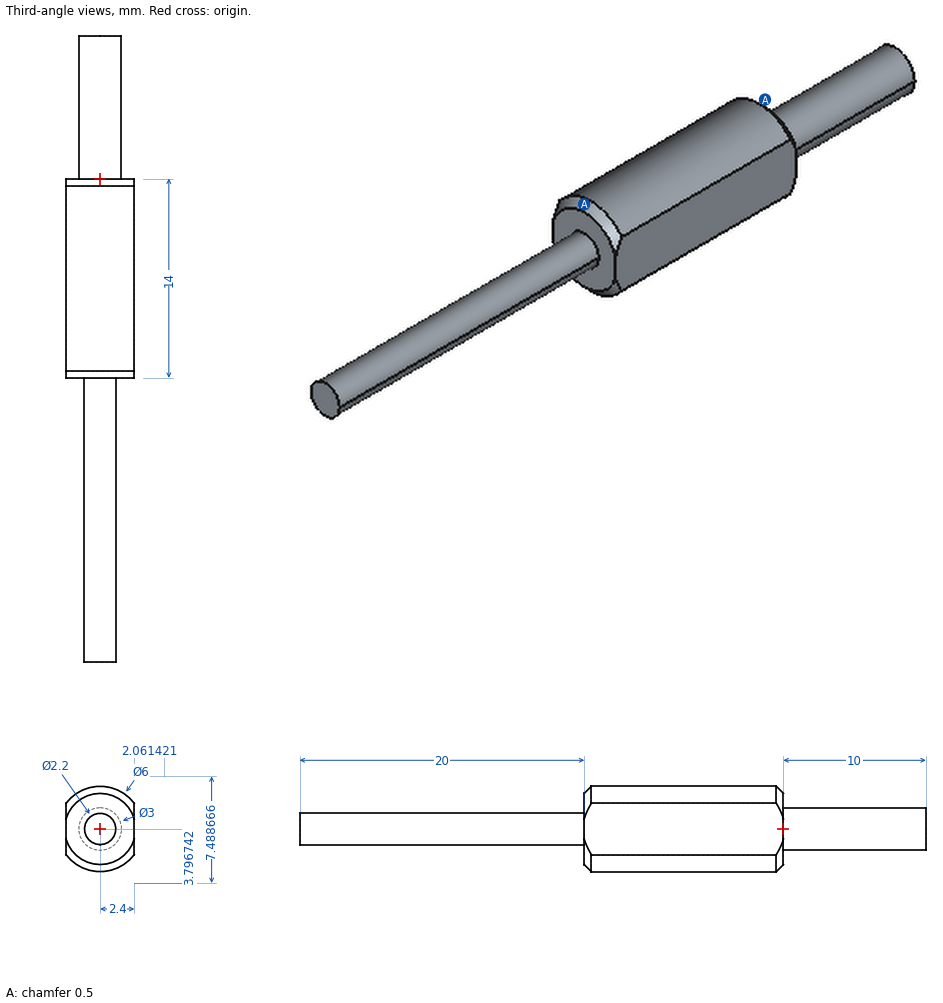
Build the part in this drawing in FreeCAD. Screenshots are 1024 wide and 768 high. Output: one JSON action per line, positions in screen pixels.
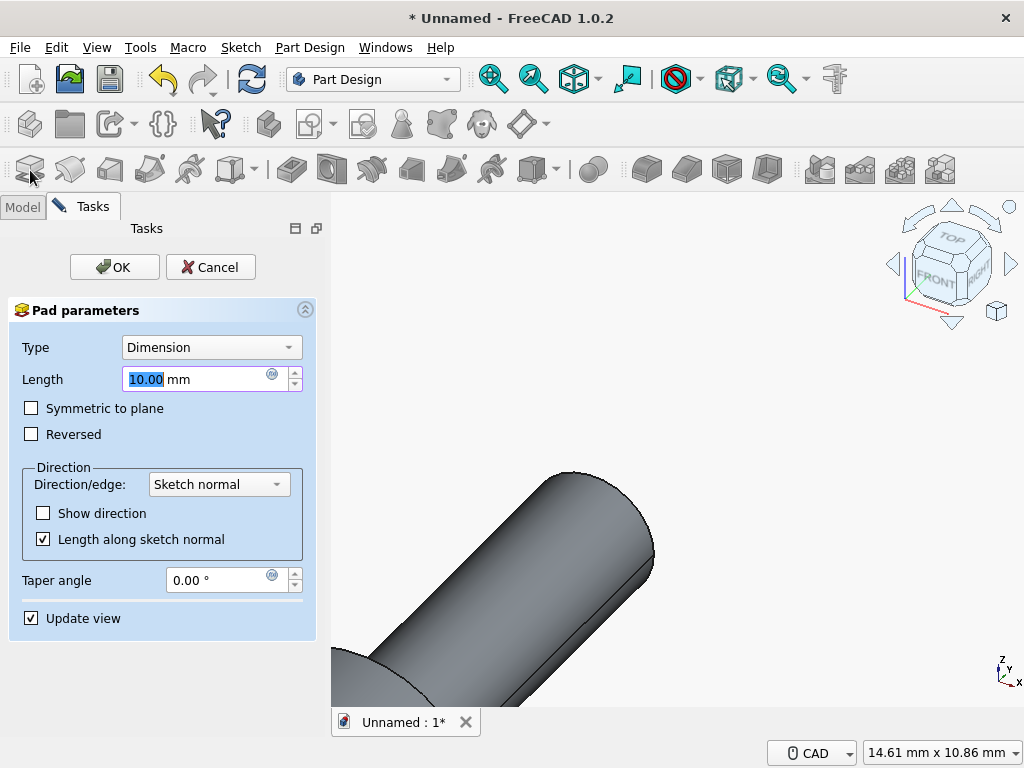
{"action": "type", "text": "14"}
{"action": "key", "text": "Tab"}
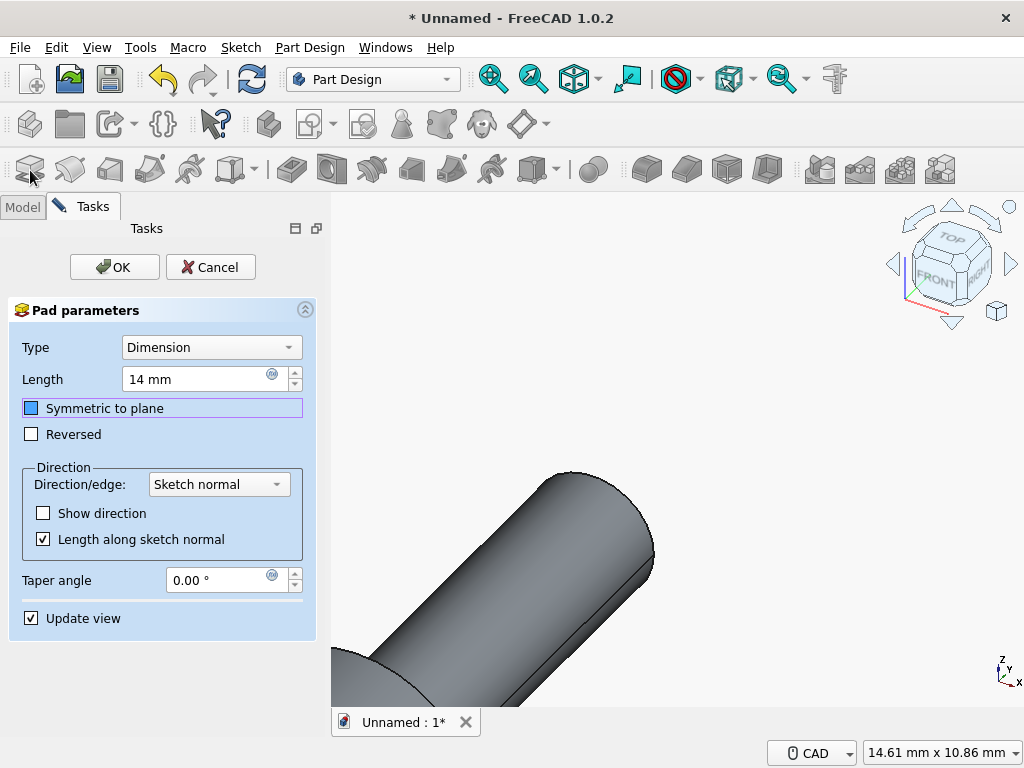
{"action": "left_click", "coordinate": [115, 267]}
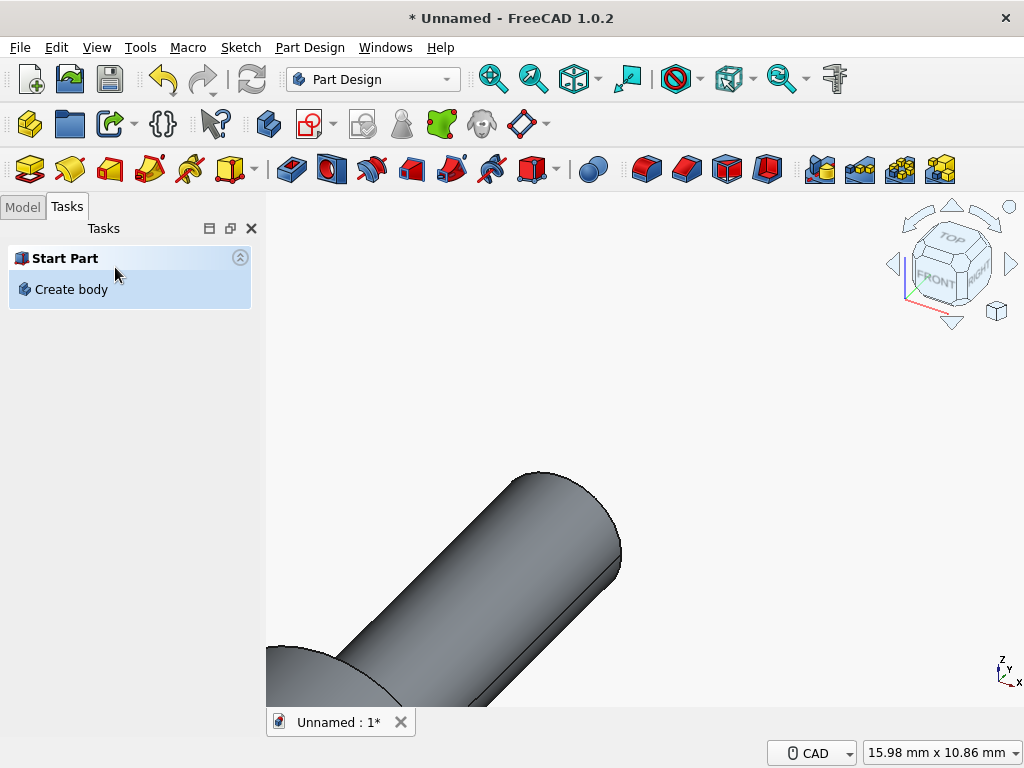
{"action": "left_click", "coordinate": [494, 80]}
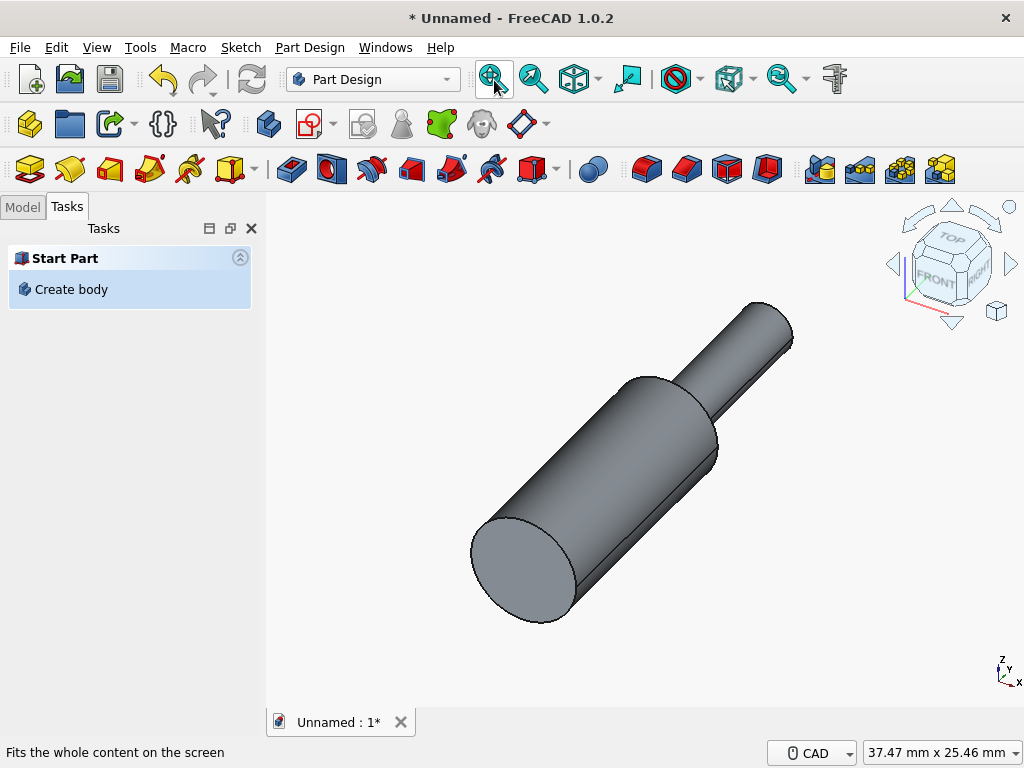
{"action": "left_click", "coordinate": [524, 569]}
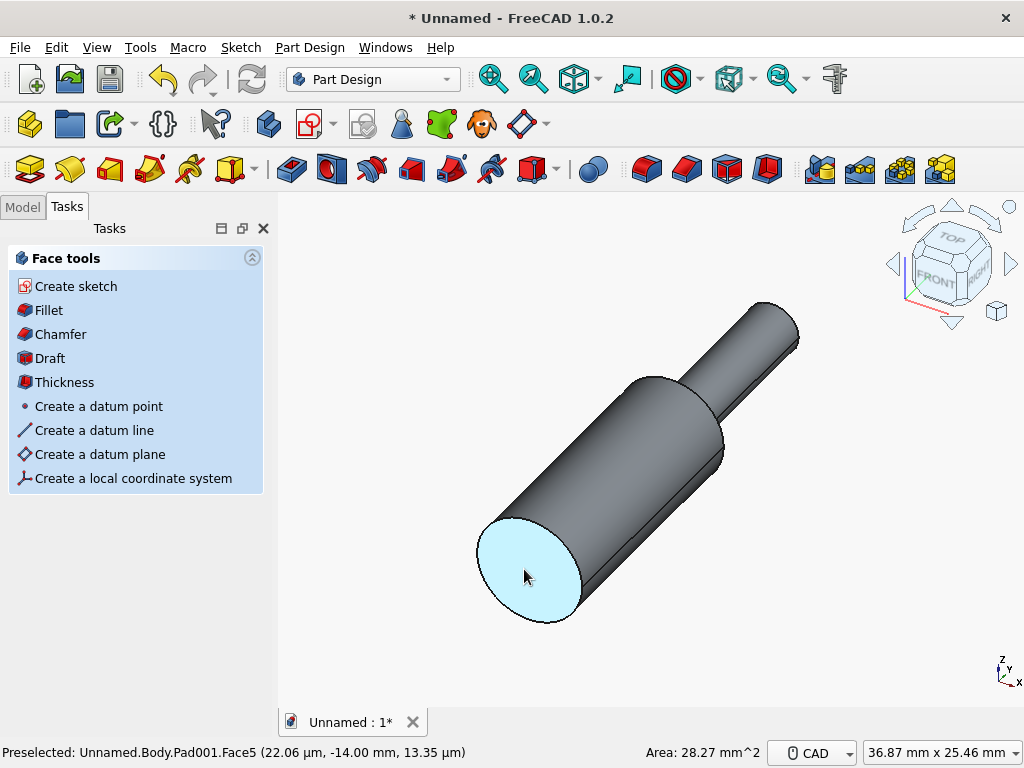
{"action": "left_click", "coordinate": [310, 124]}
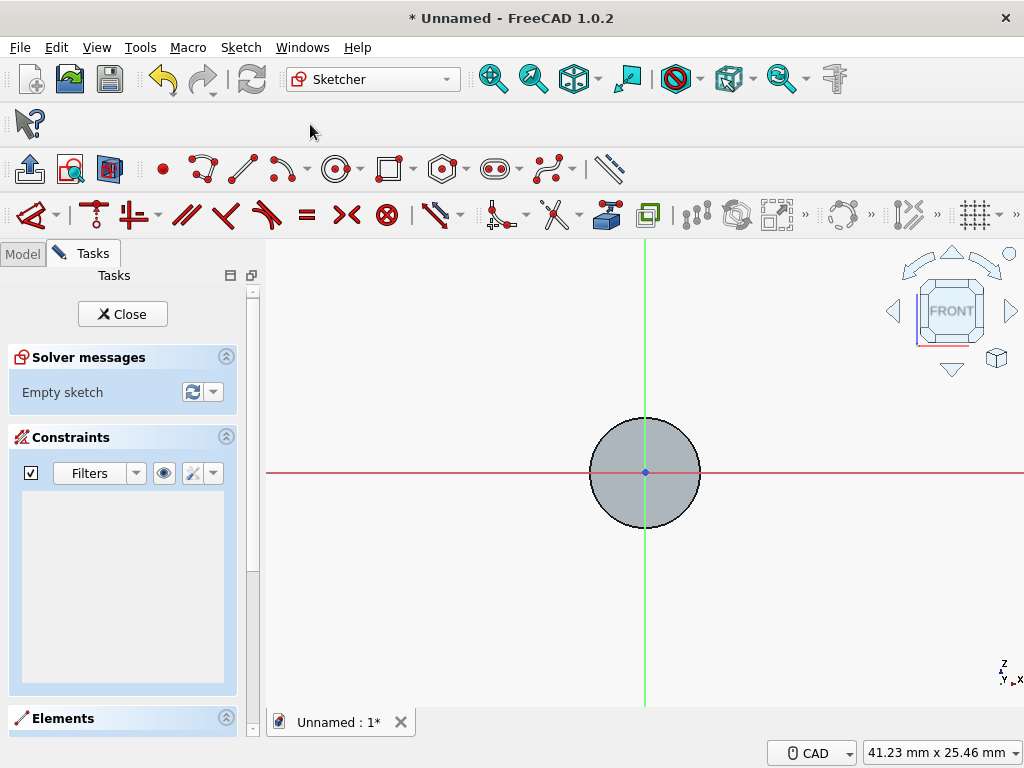
{"action": "scroll", "coordinate": [656, 473], "scroll_direction": "up", "scroll_amount": 10}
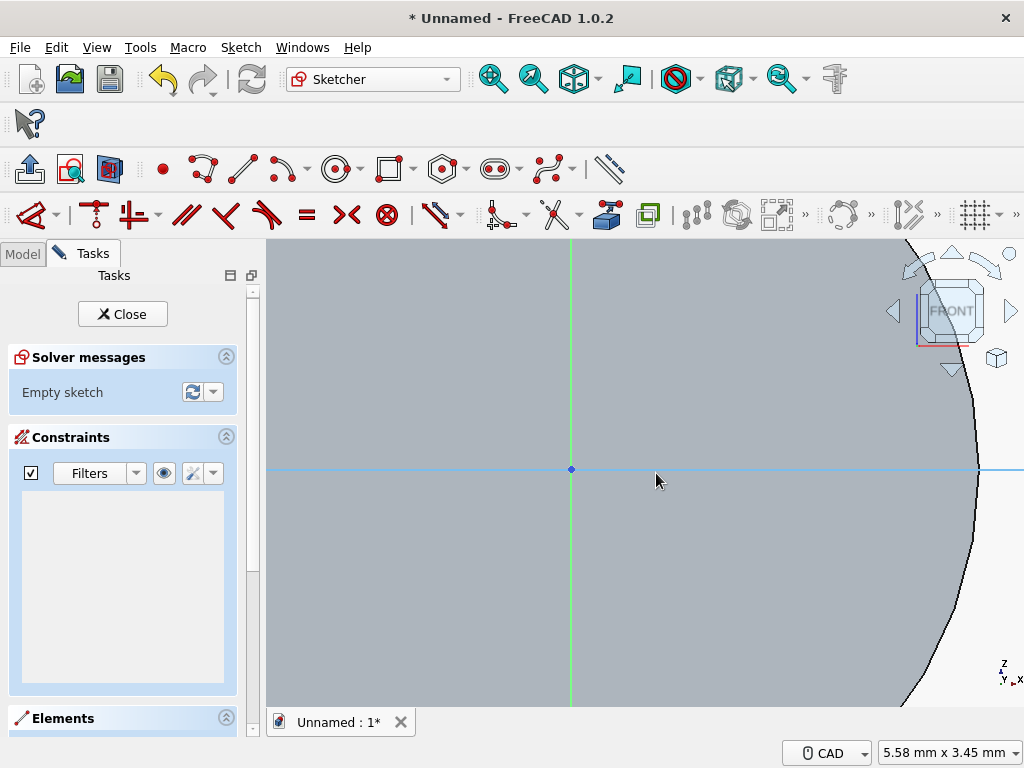
{"action": "left_click", "coordinate": [336, 170]}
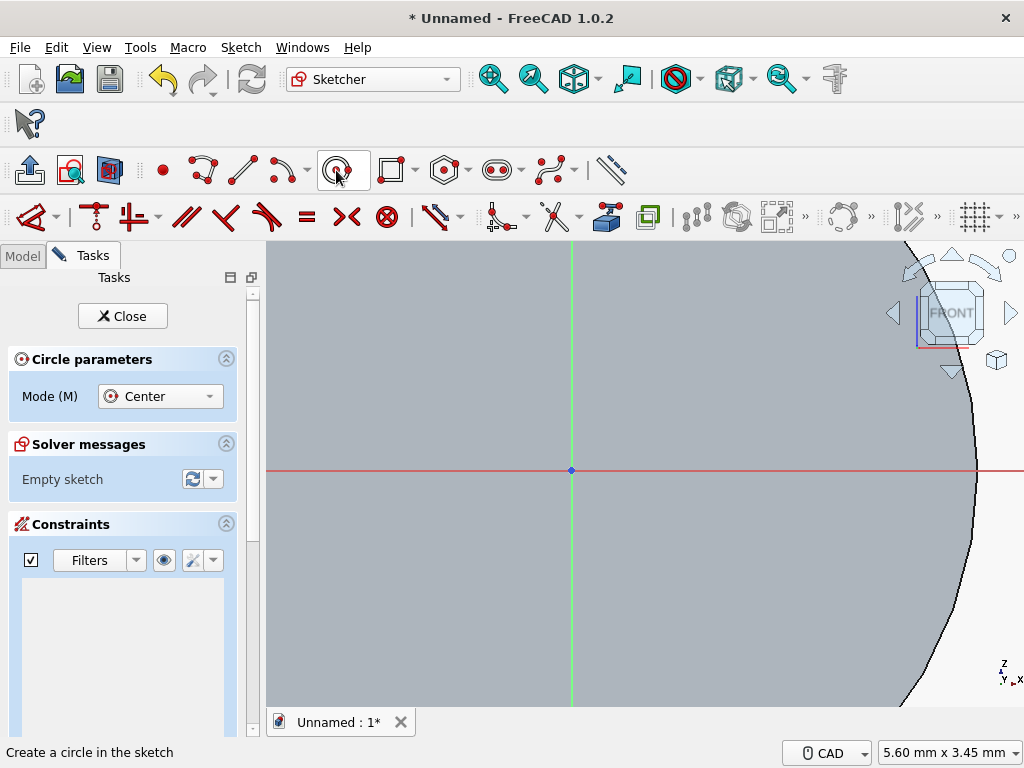
{"action": "left_click", "coordinate": [572, 471]}
{"action": "left_click", "coordinate": [677, 366]}
{"action": "key", "text": "Escape"}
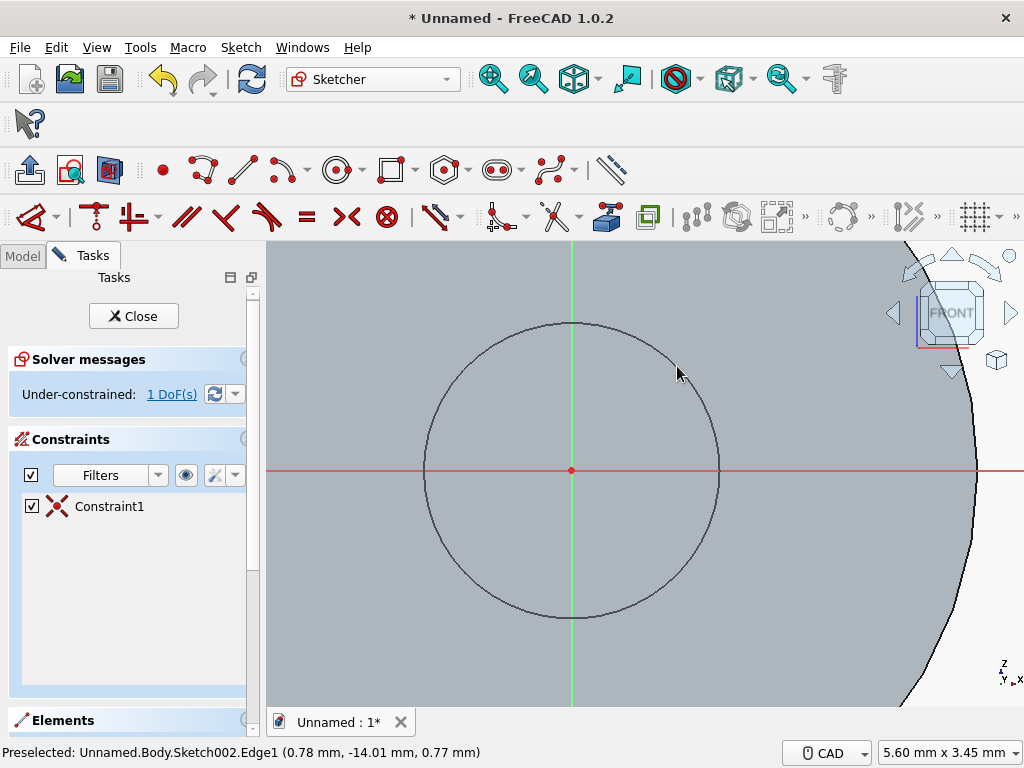
{"action": "left_click", "coordinate": [32, 218]}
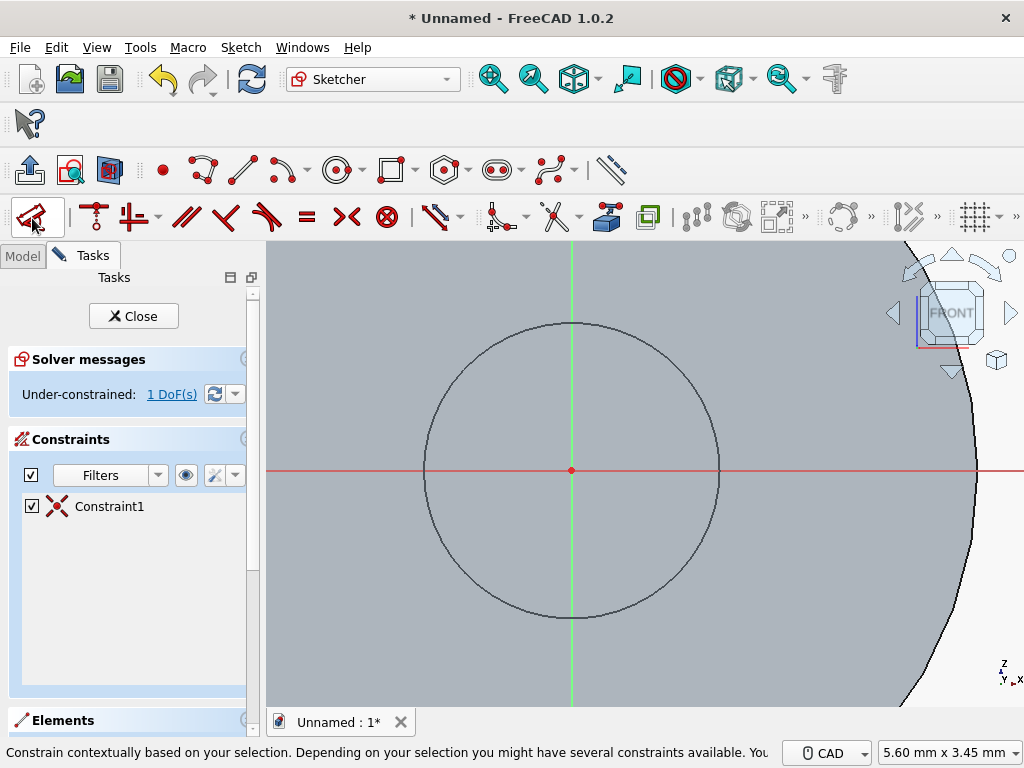
{"action": "left_click", "coordinate": [676, 366]}
{"action": "left_click", "coordinate": [699, 343]}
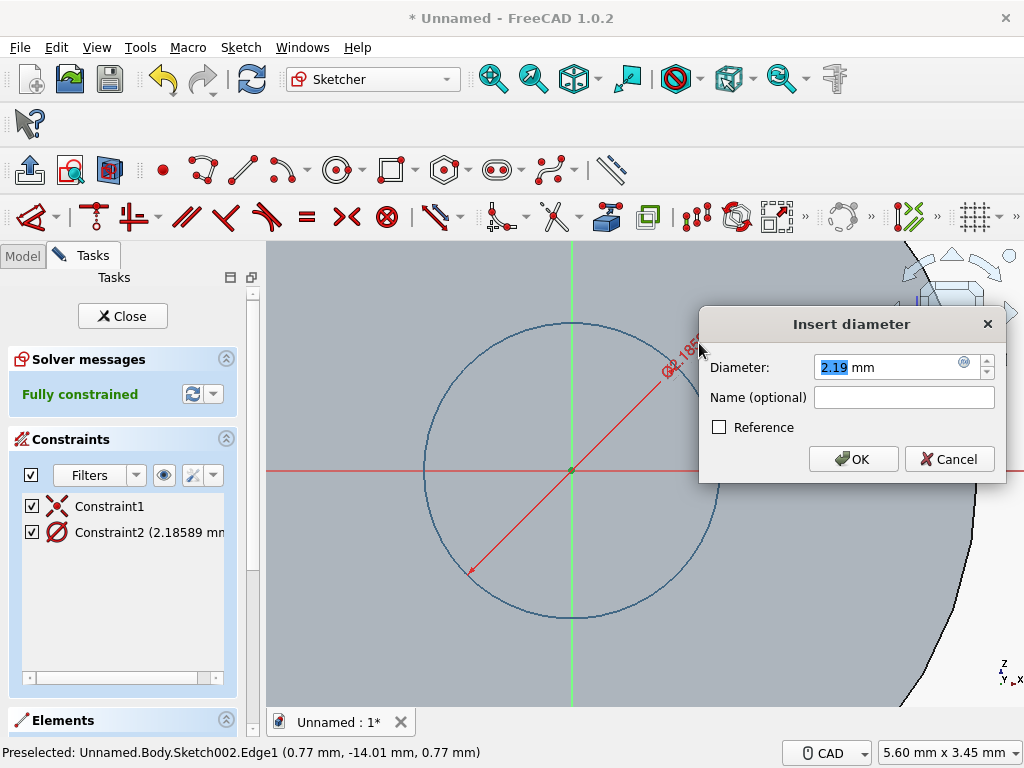
{"action": "type", "text": "2.2"}
{"action": "key", "text": "Return"}
{"action": "key", "text": "Escape"}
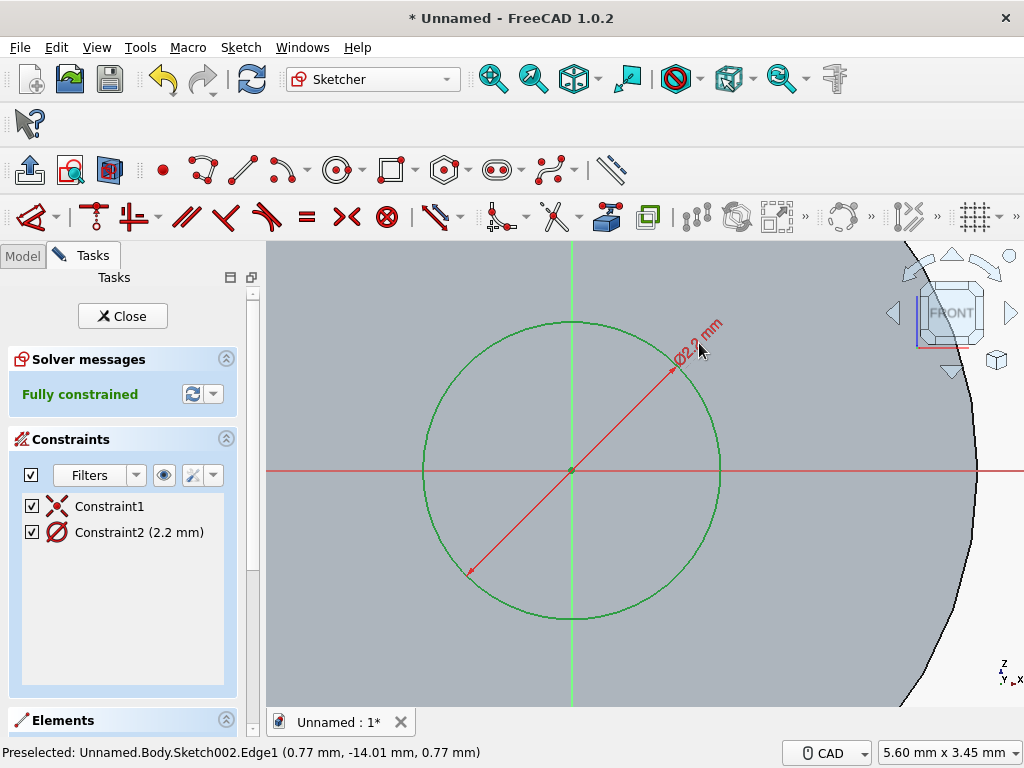
{"action": "left_click", "coordinate": [123, 316]}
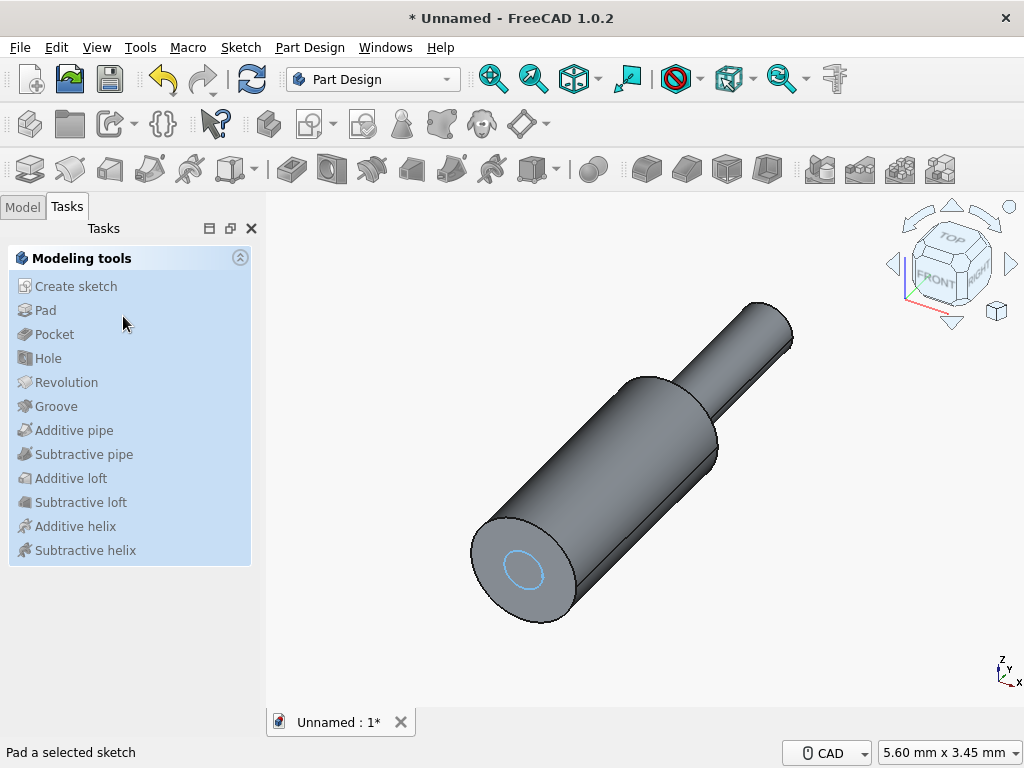
{"action": "left_click", "coordinate": [30, 170]}